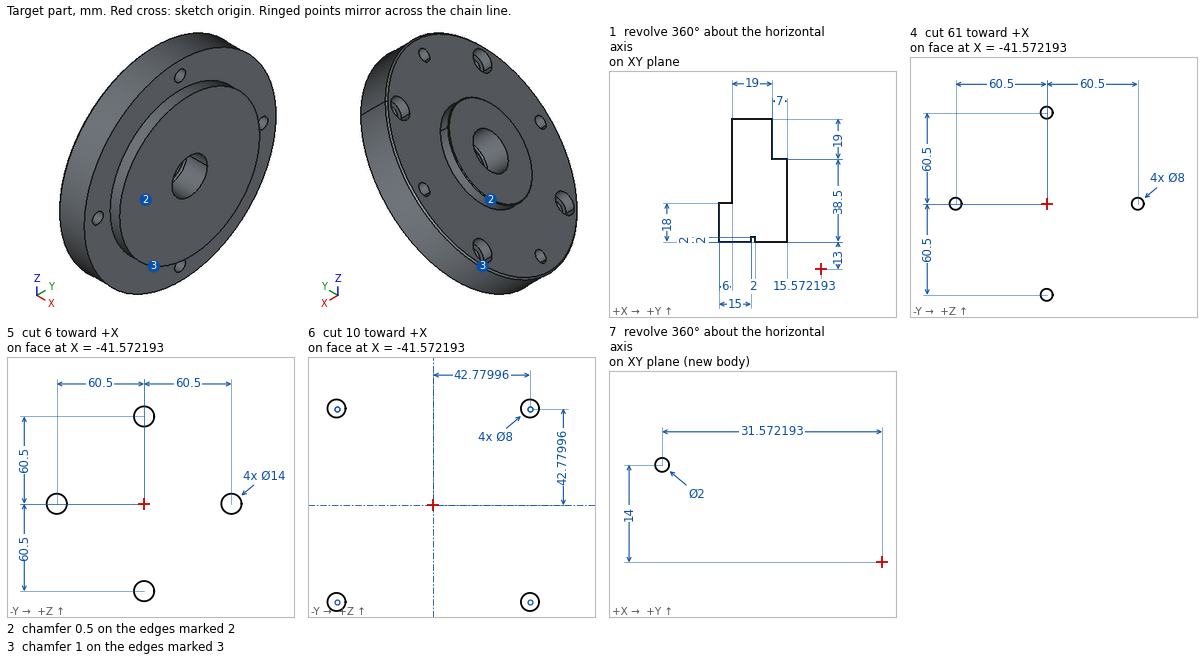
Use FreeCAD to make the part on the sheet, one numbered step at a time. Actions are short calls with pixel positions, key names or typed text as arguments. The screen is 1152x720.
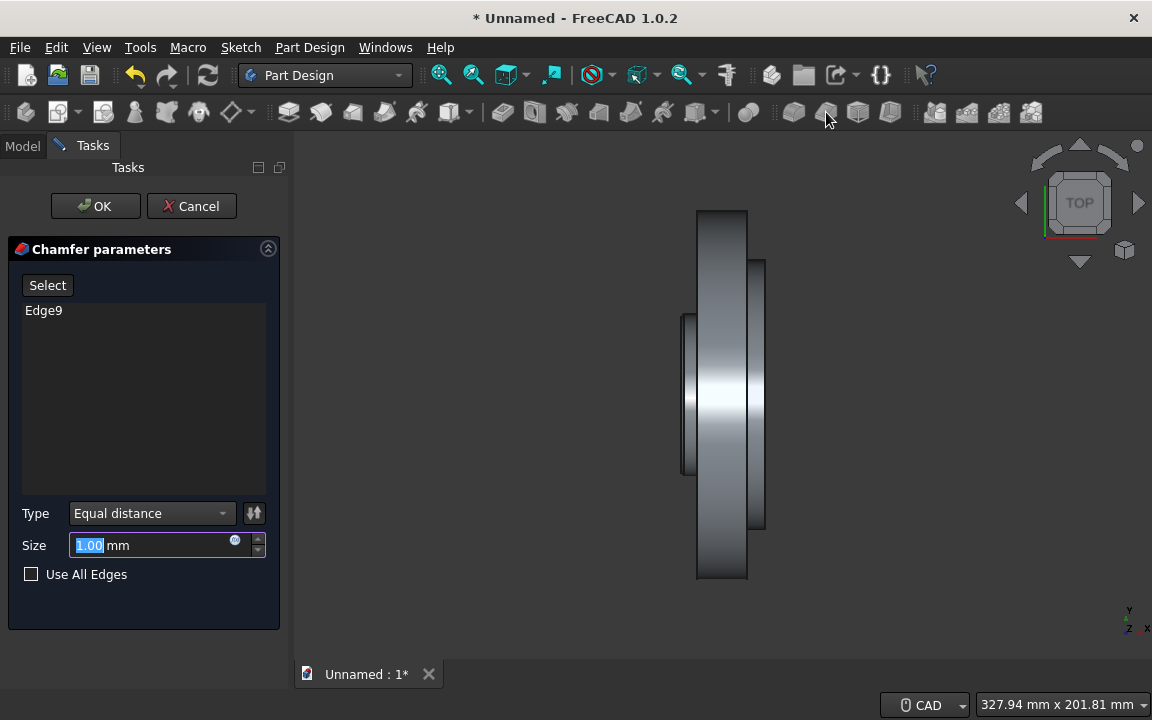
text(0.5)
key(Tab)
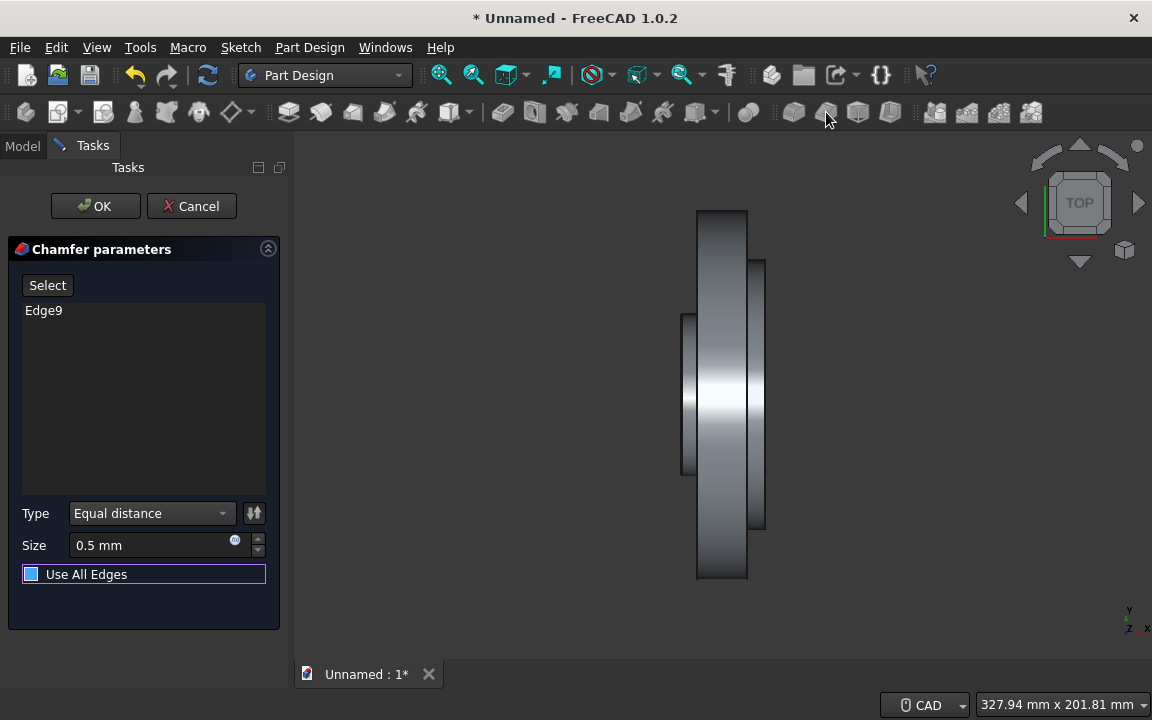
click(96, 206)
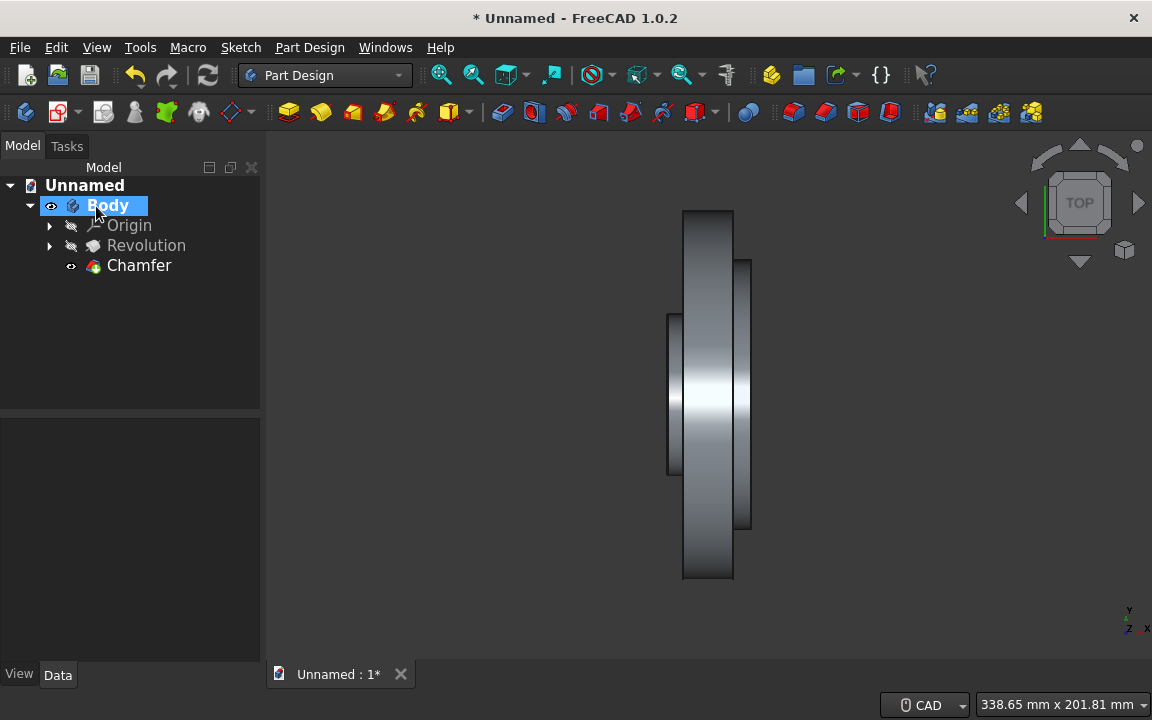
click(683, 543)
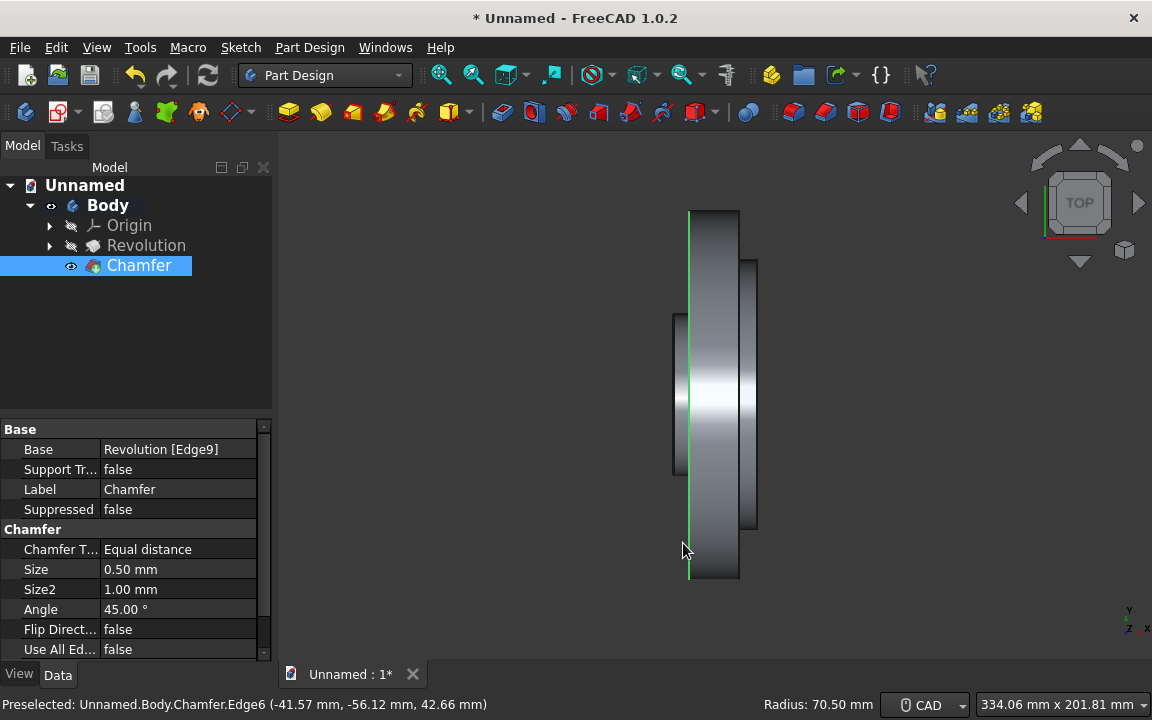
click(826, 112)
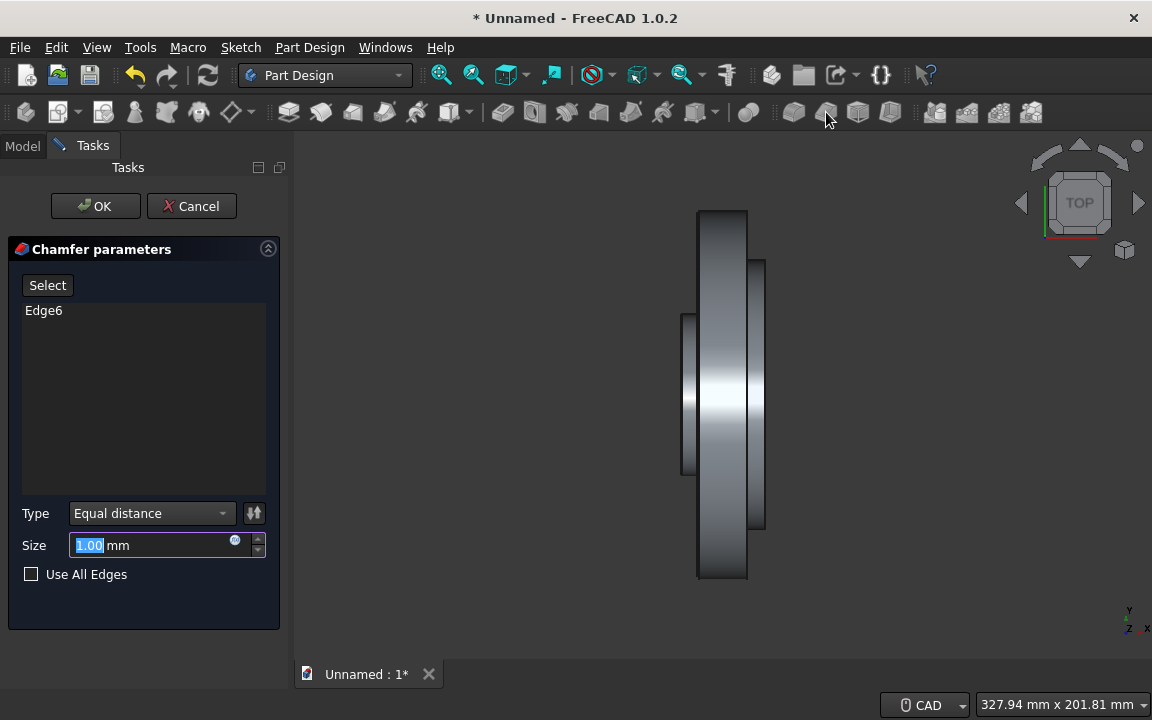
text(1)
key(Tab)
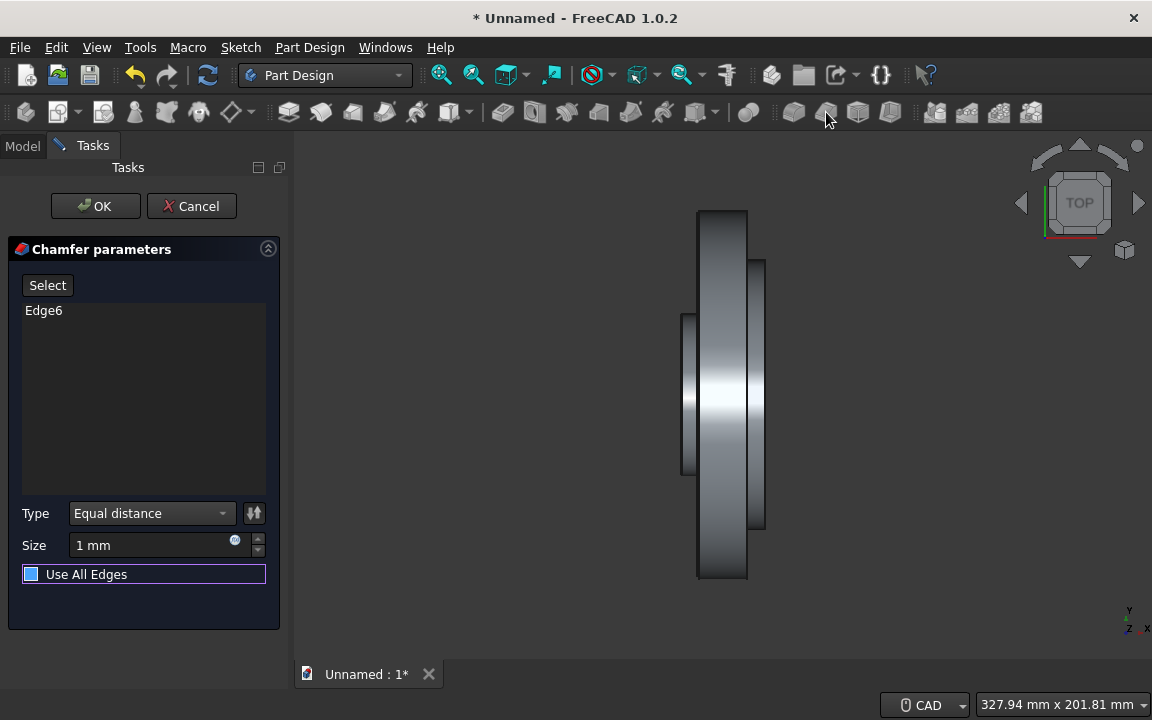
click(96, 206)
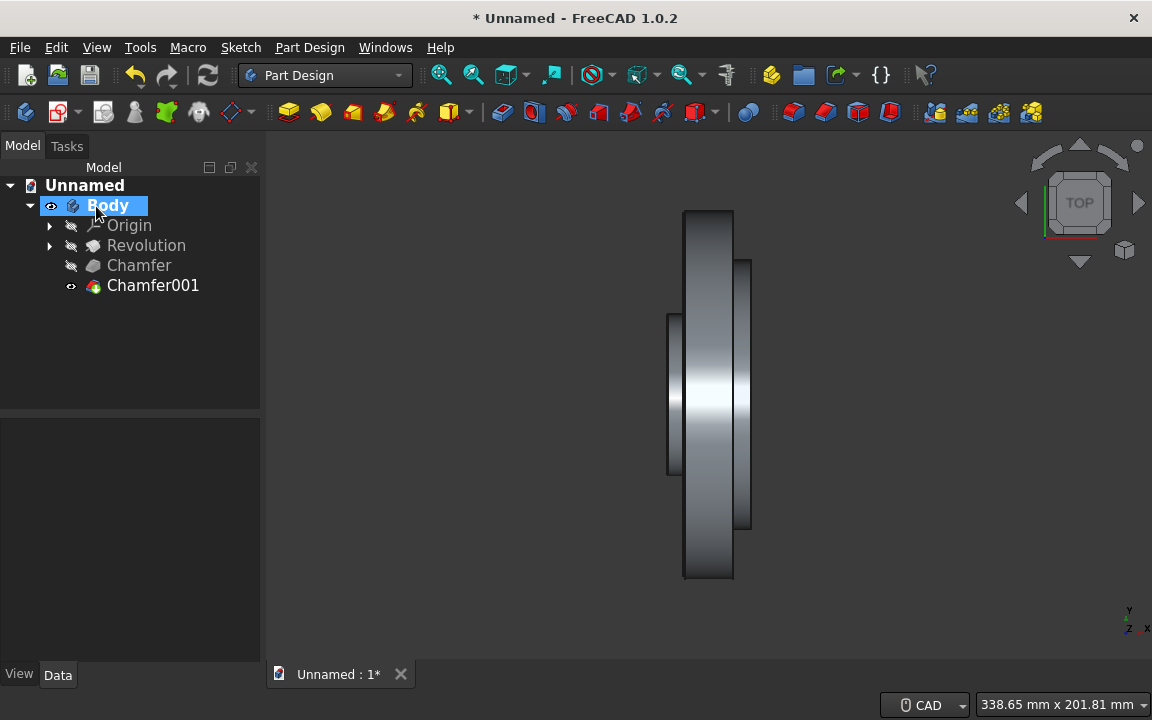
key(6)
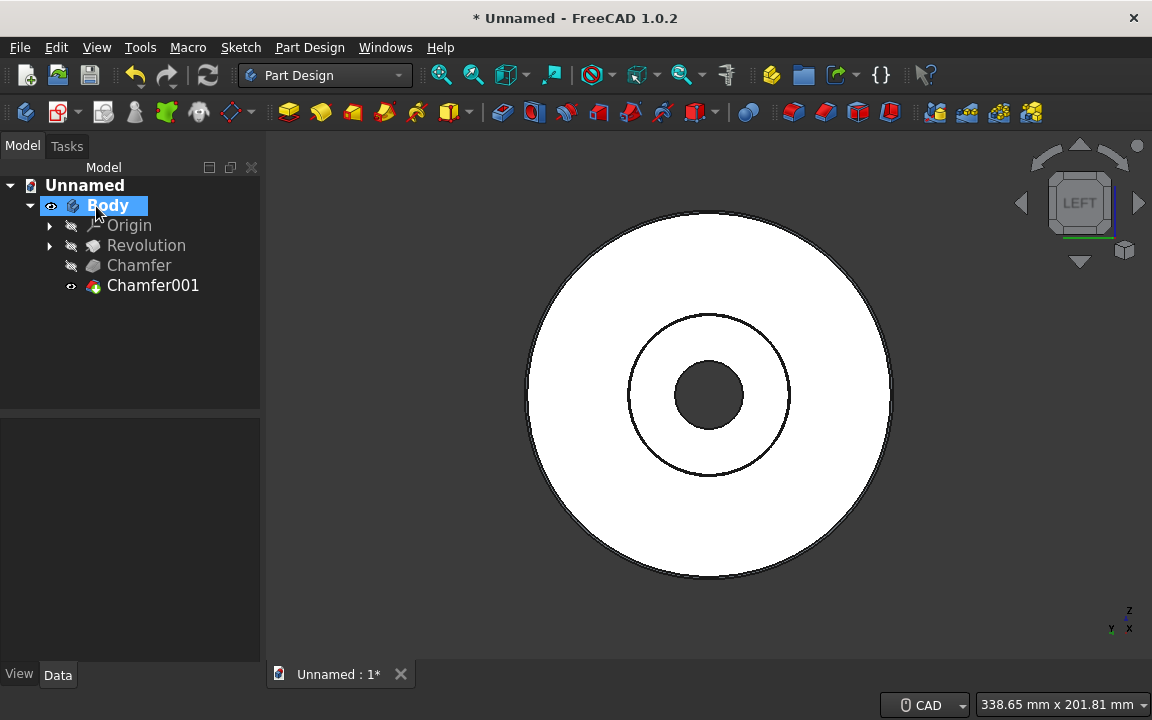
click(657, 498)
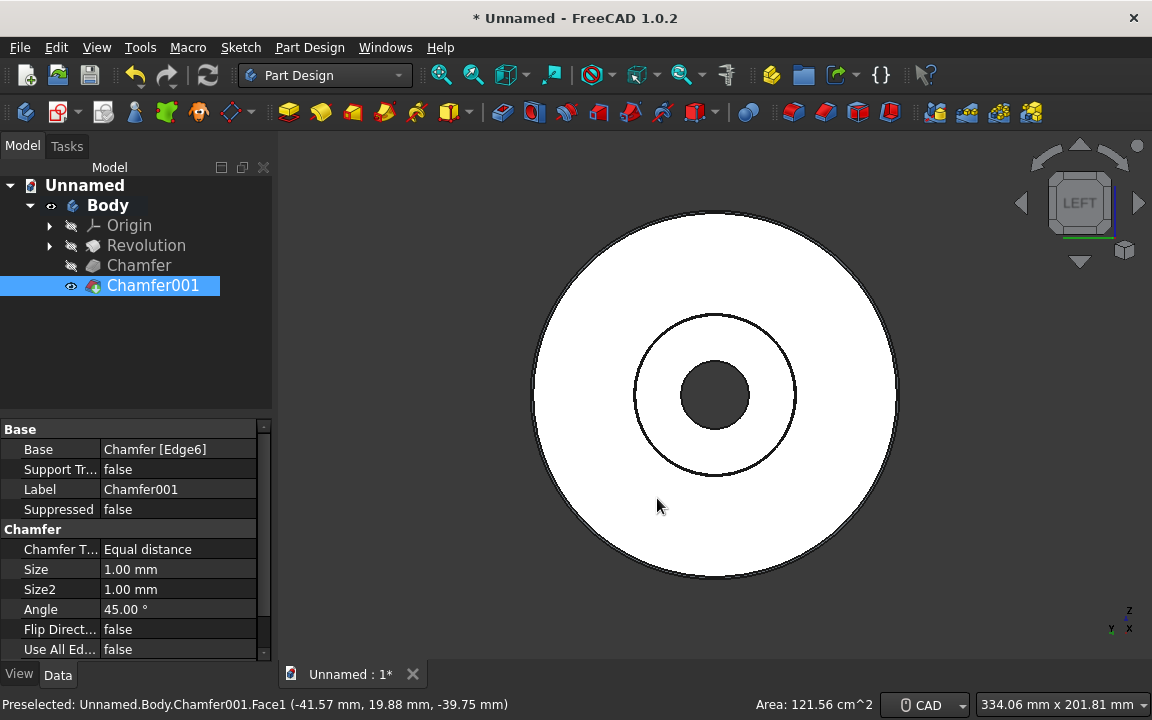
click(58, 112)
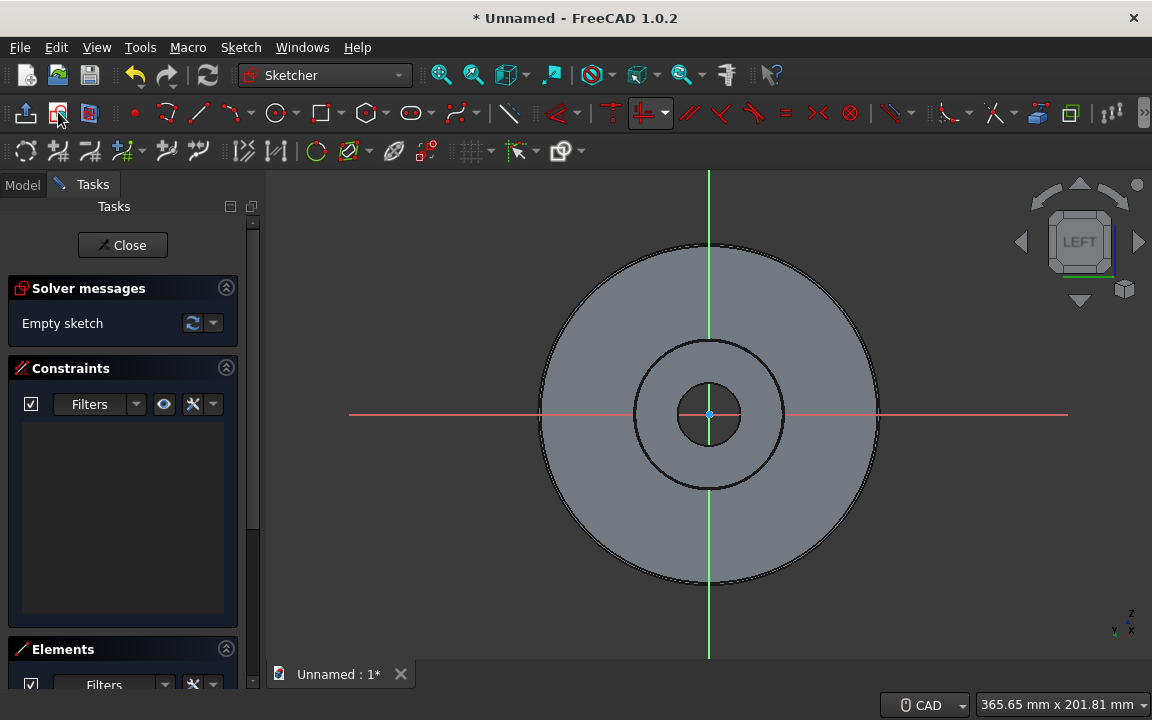
click(90, 114)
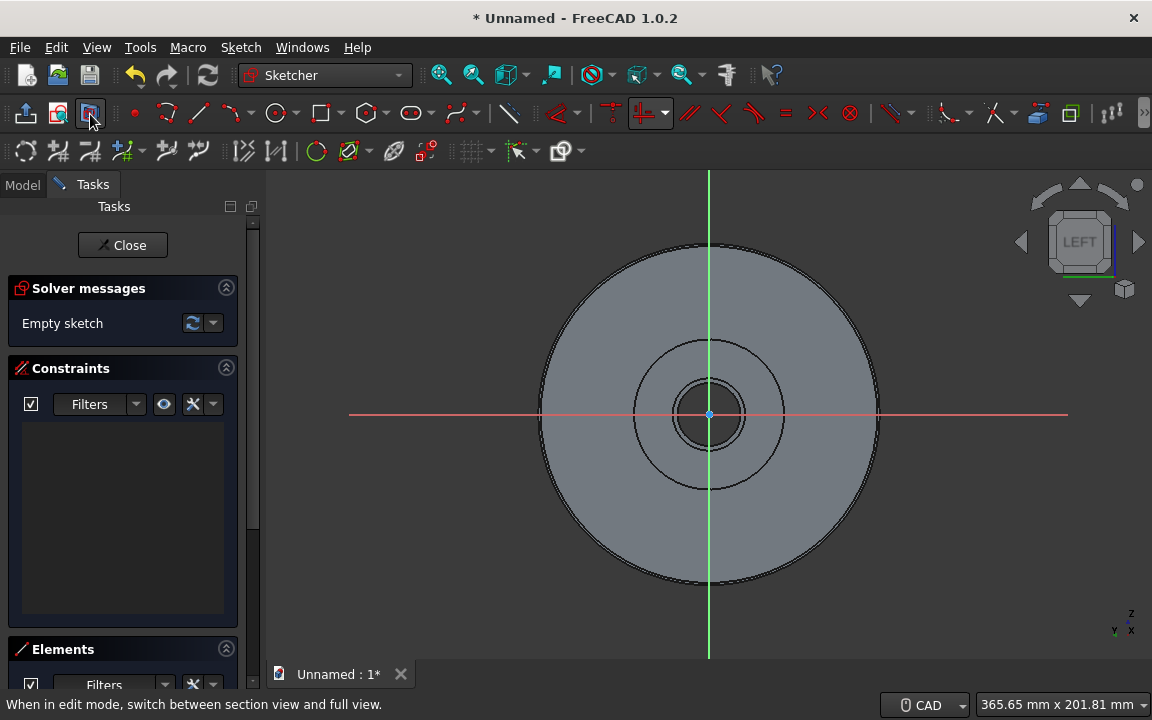
click(276, 114)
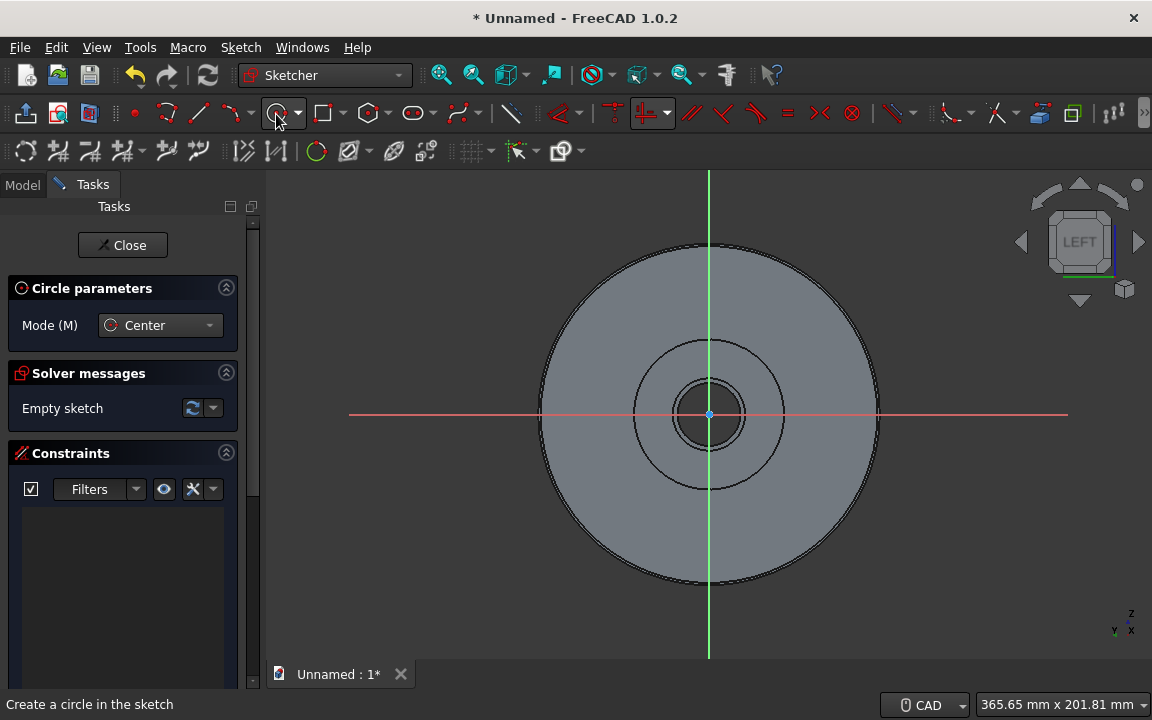
scroll(856, 414, up, 5)